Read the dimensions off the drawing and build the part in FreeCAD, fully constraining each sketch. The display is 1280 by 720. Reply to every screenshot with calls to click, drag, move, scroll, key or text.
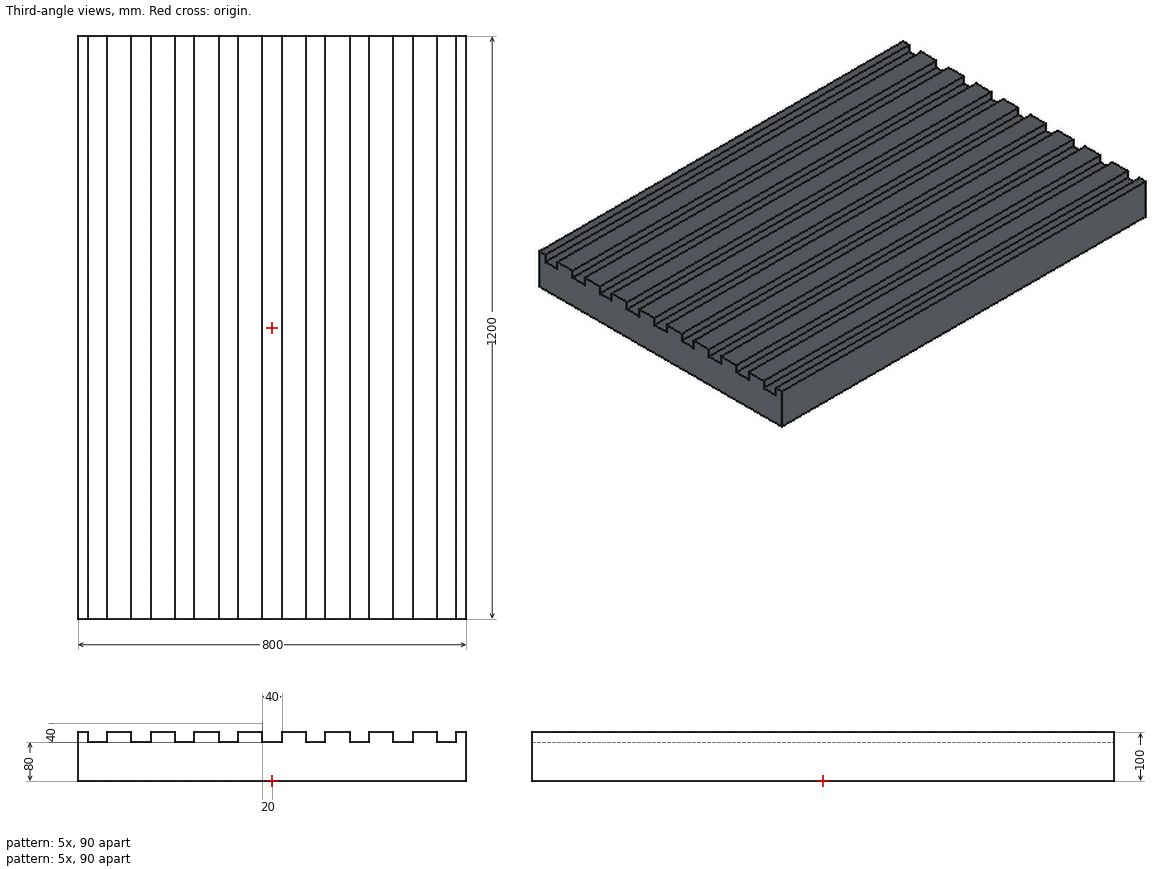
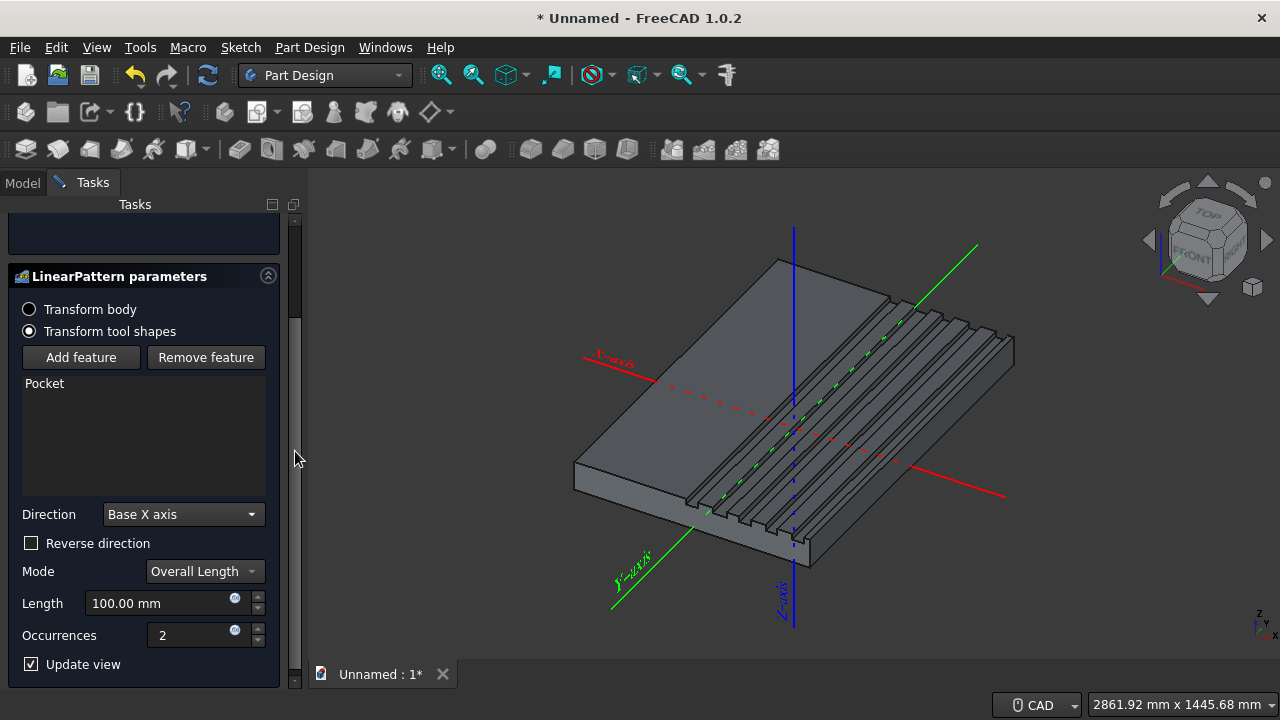
click(206, 572)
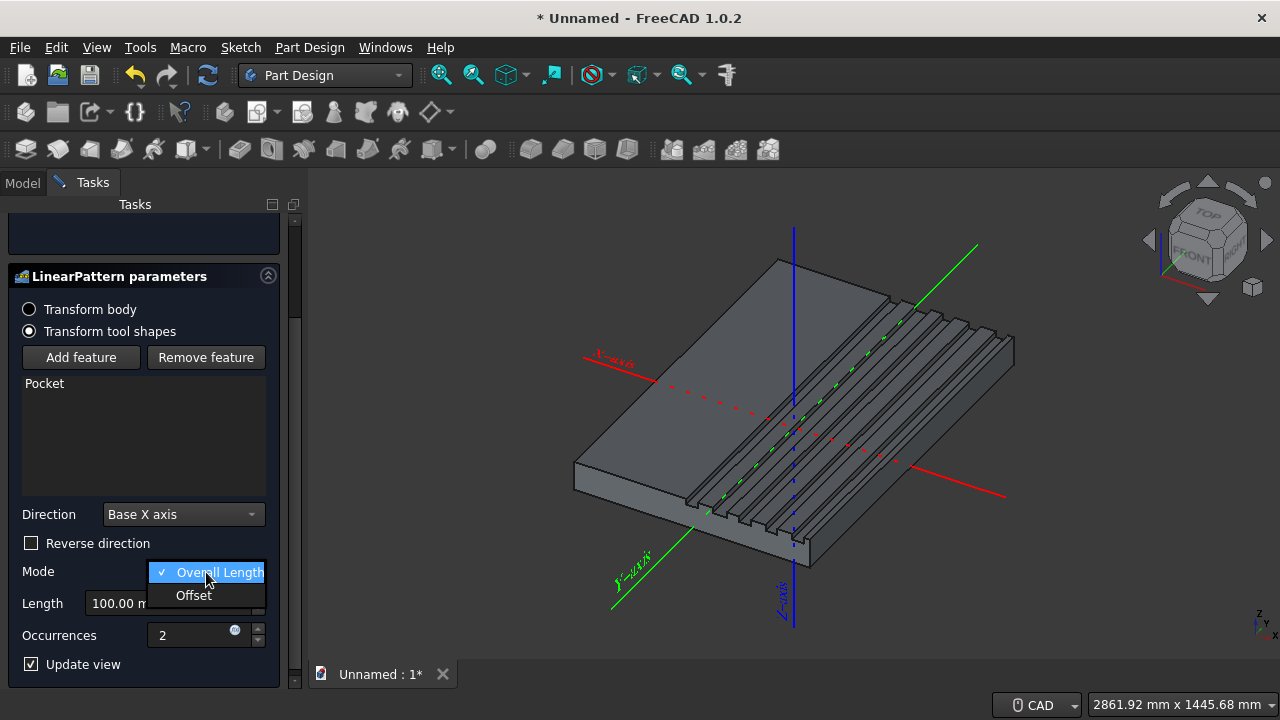
click(206, 596)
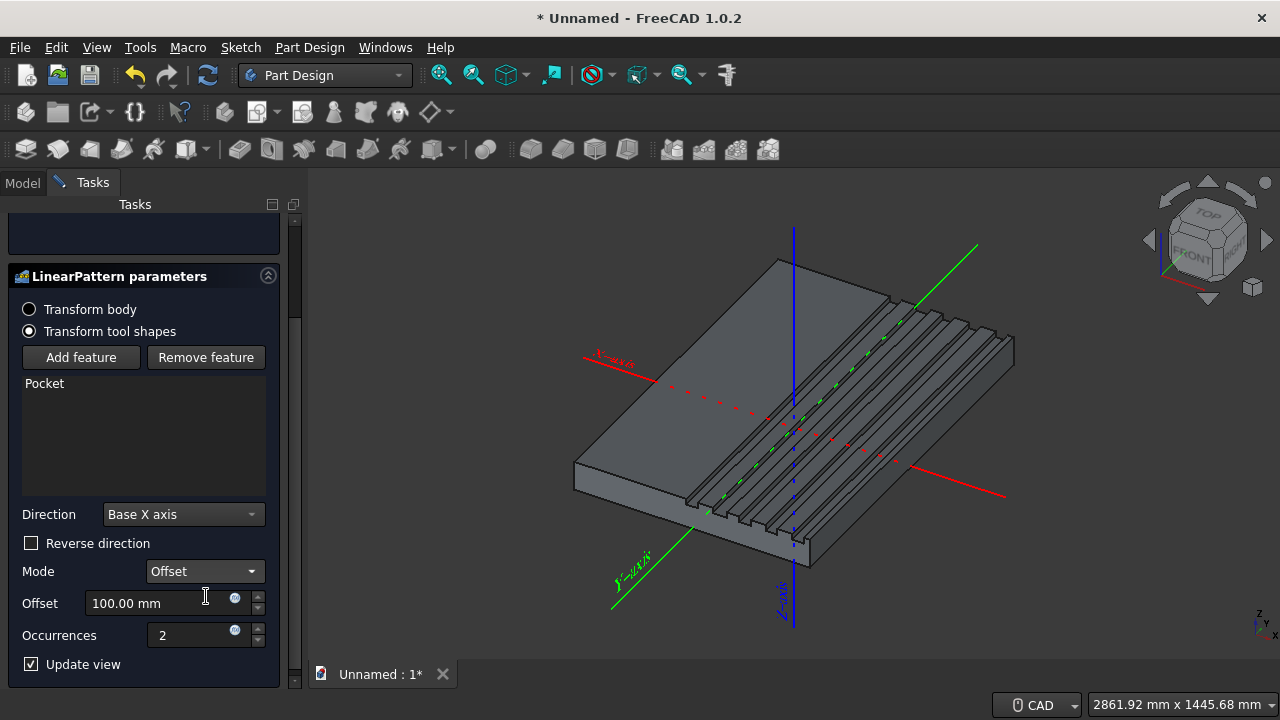
triple_click(168, 603)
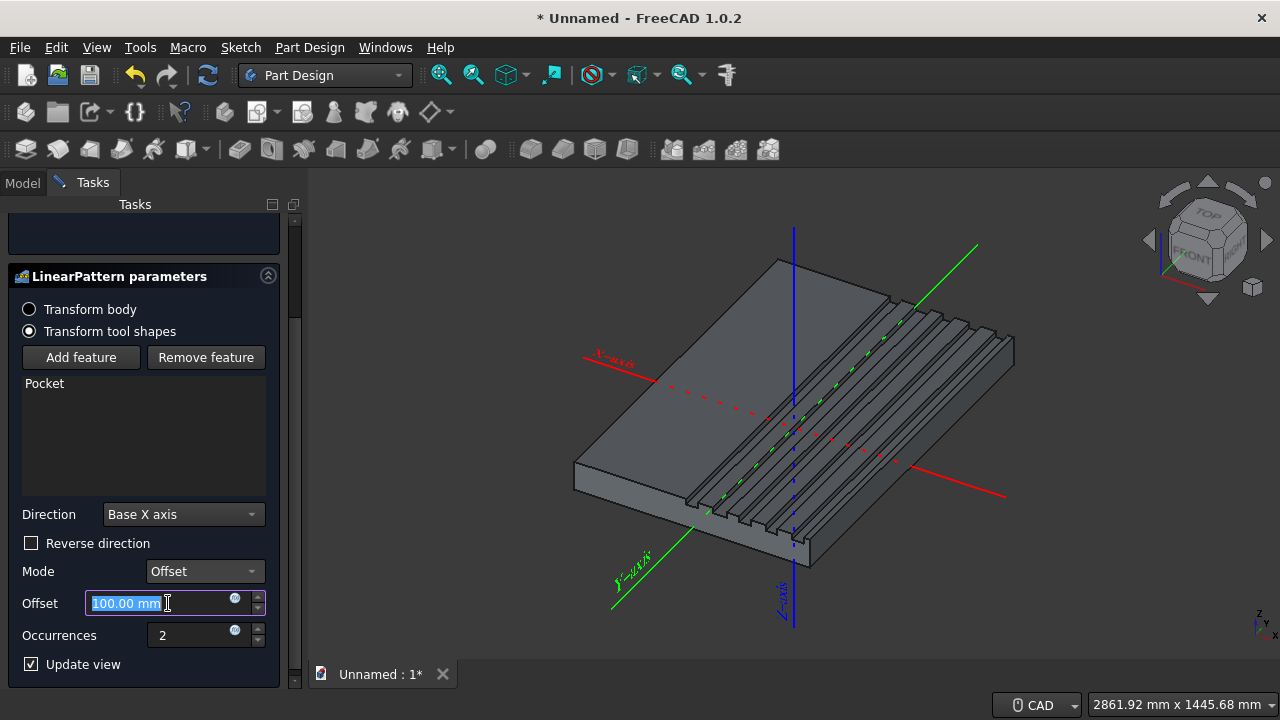
text(90)
key(Tab)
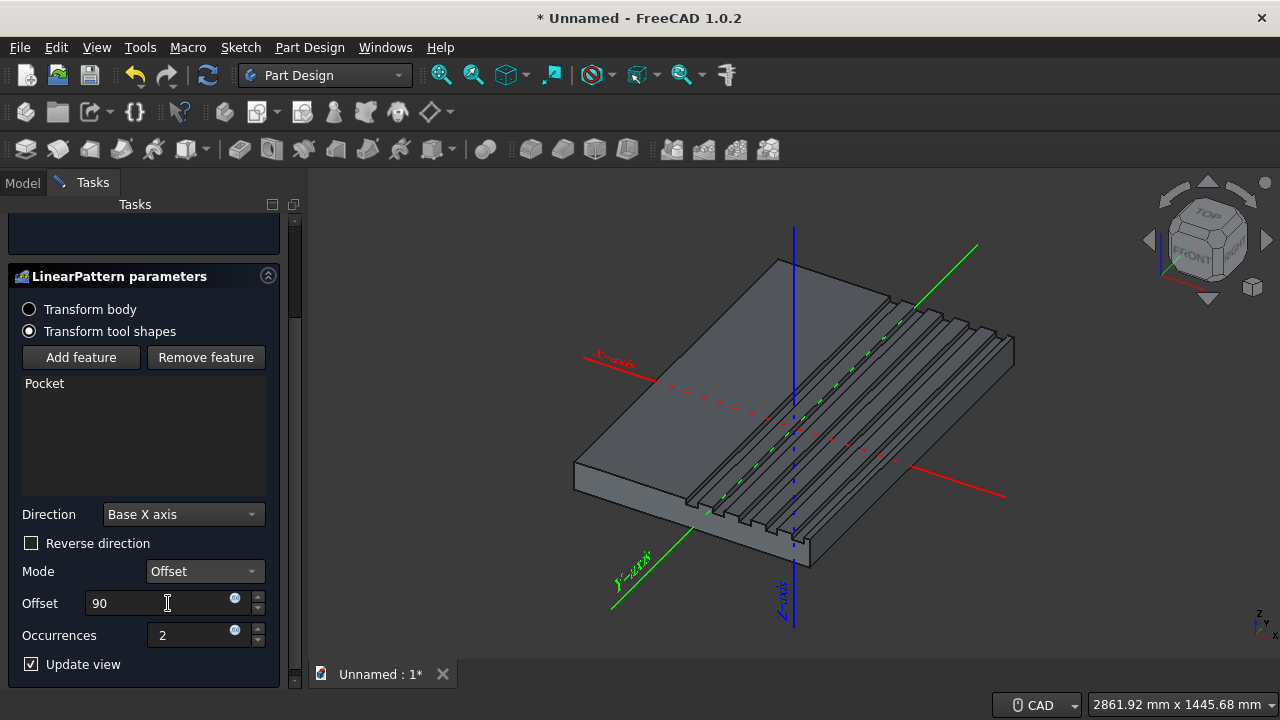
triple_click(198, 635)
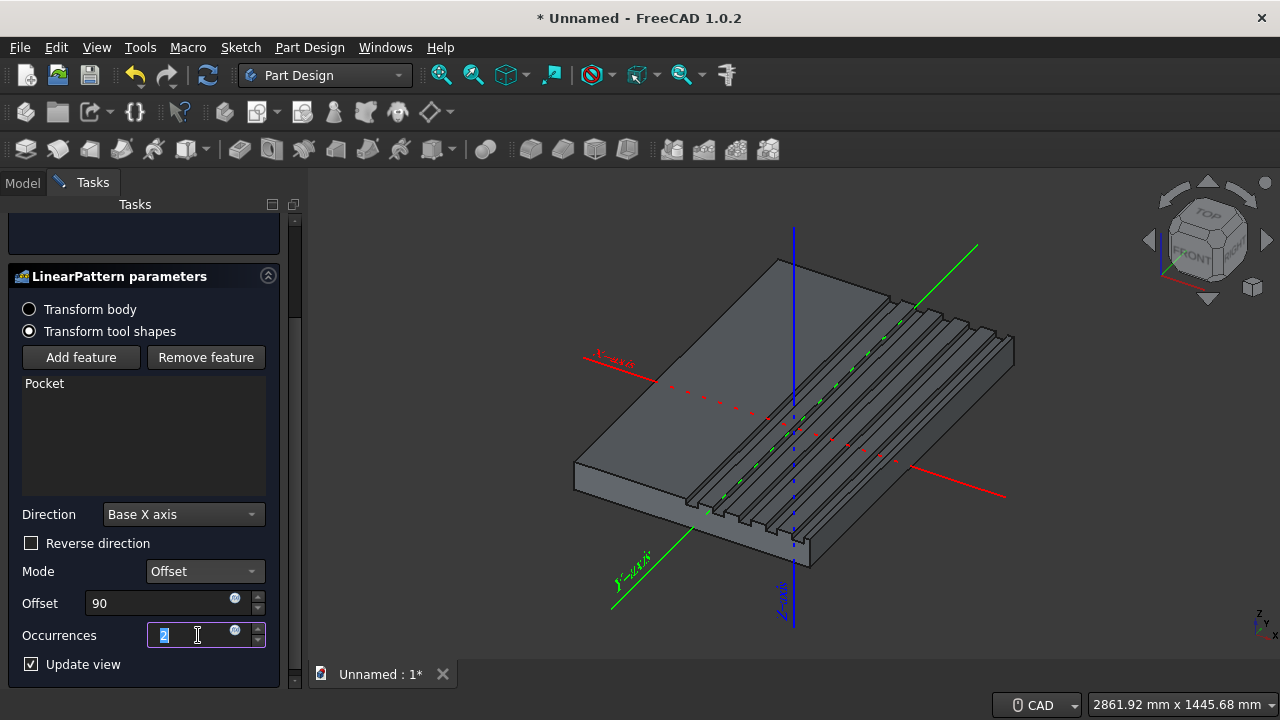
text(5)
key(Tab)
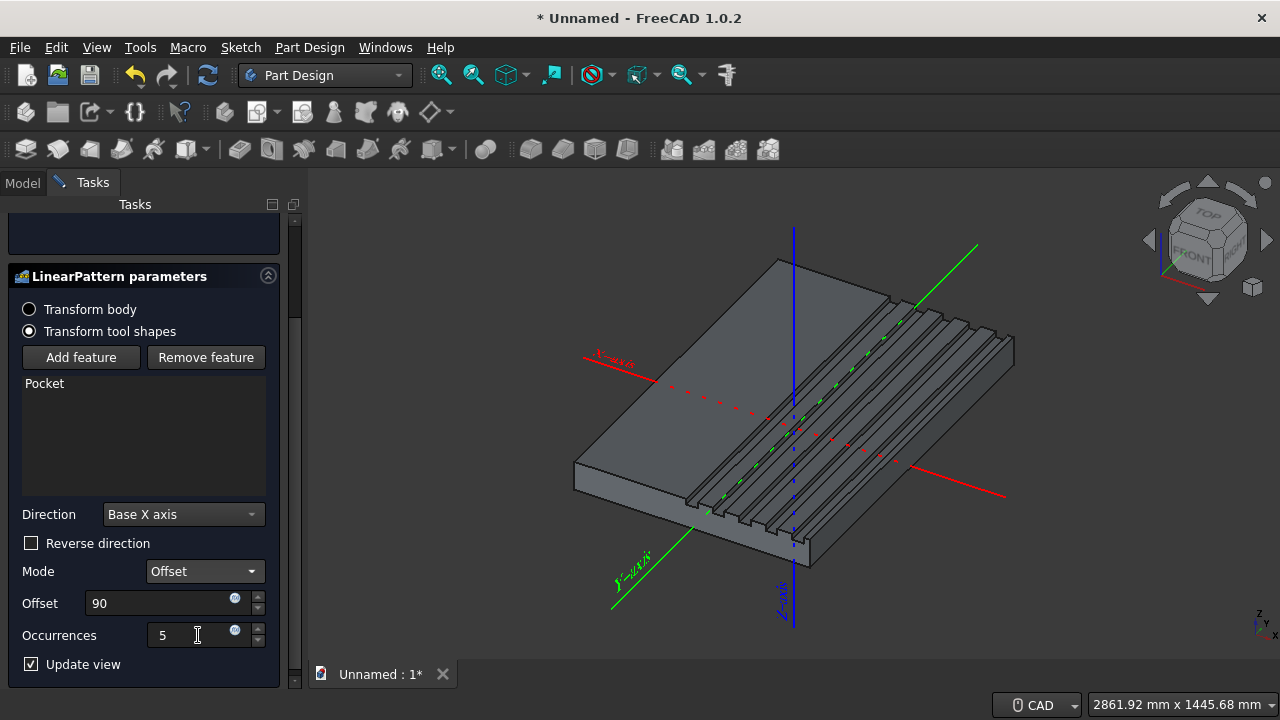
click(30, 543)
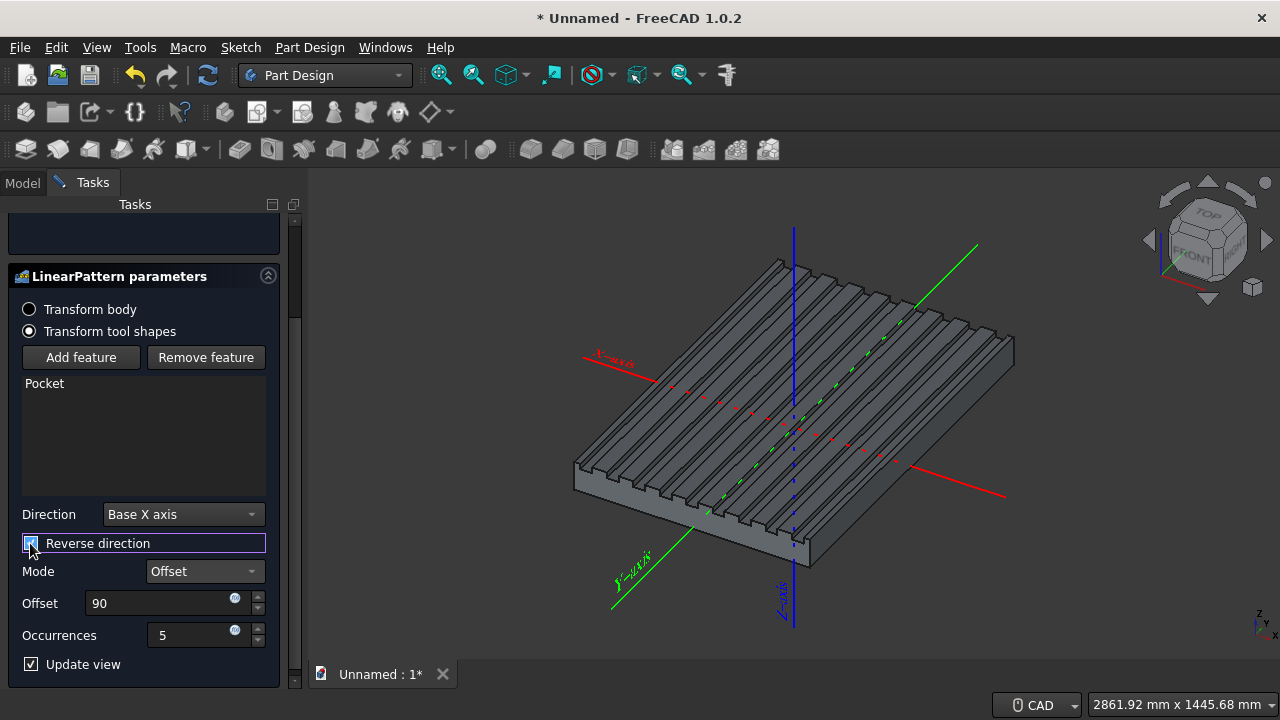
scroll(295, 451, up, 3)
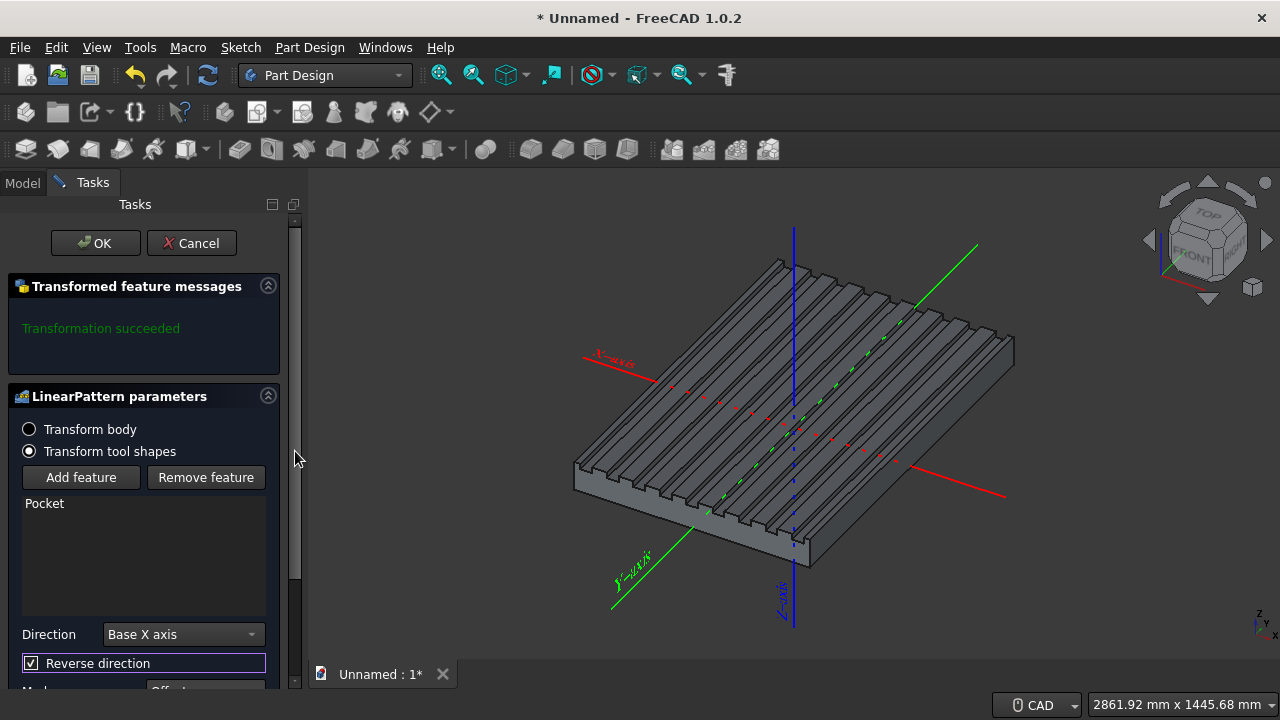
click(96, 243)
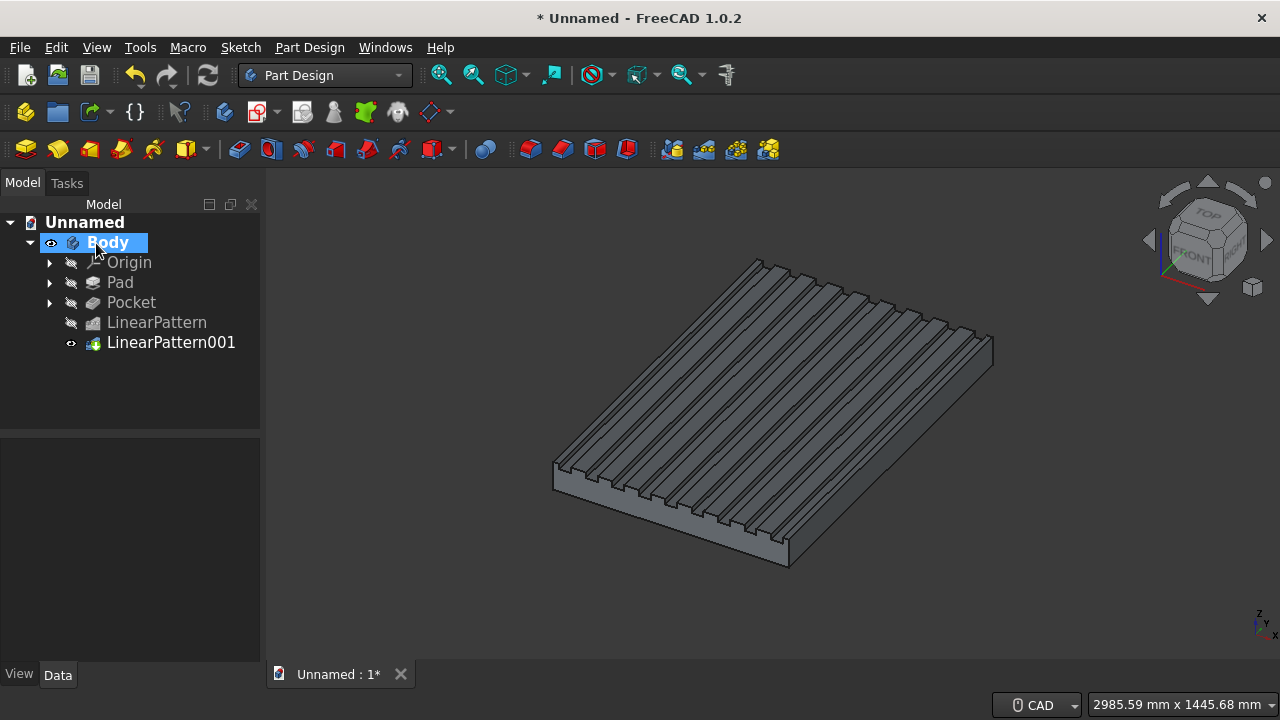
key(0)